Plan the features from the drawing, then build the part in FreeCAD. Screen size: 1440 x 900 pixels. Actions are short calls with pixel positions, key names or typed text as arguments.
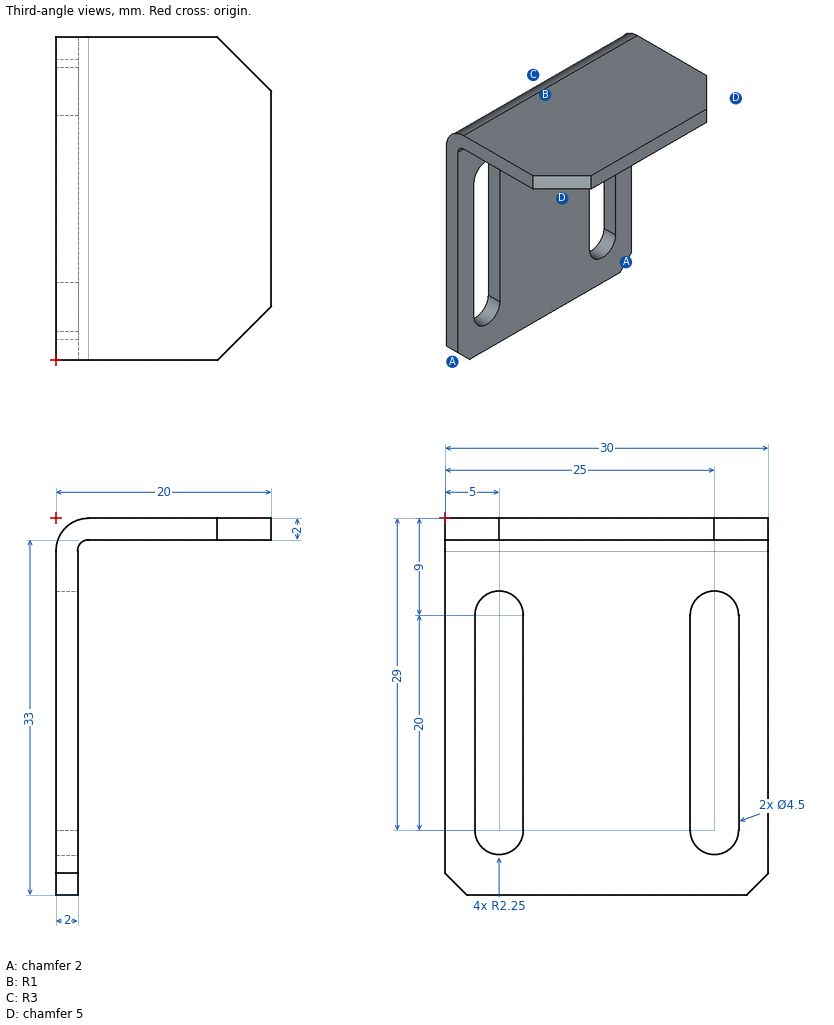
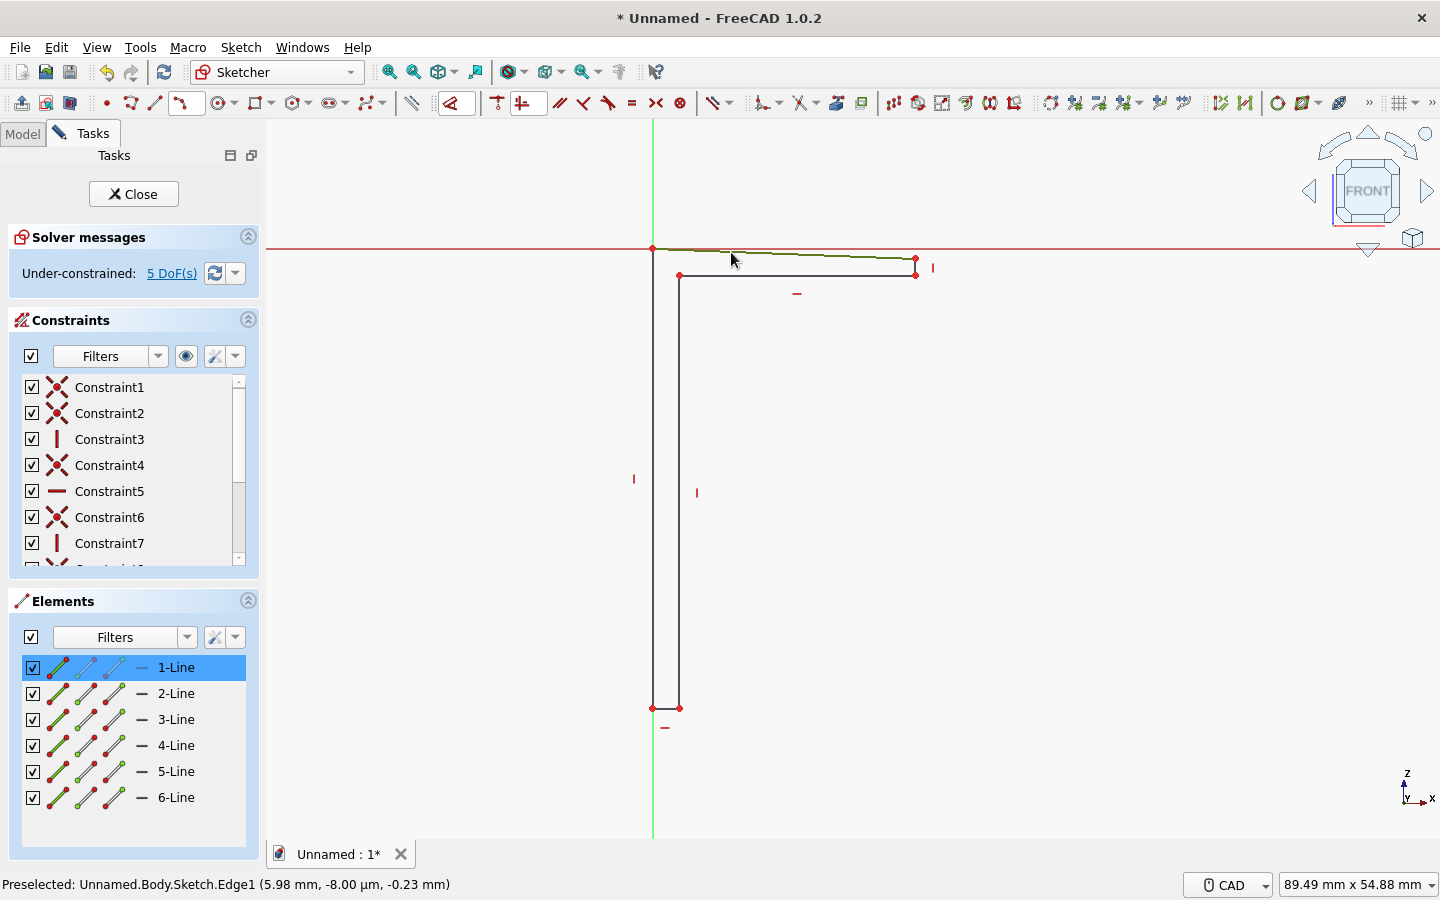
click(542, 104)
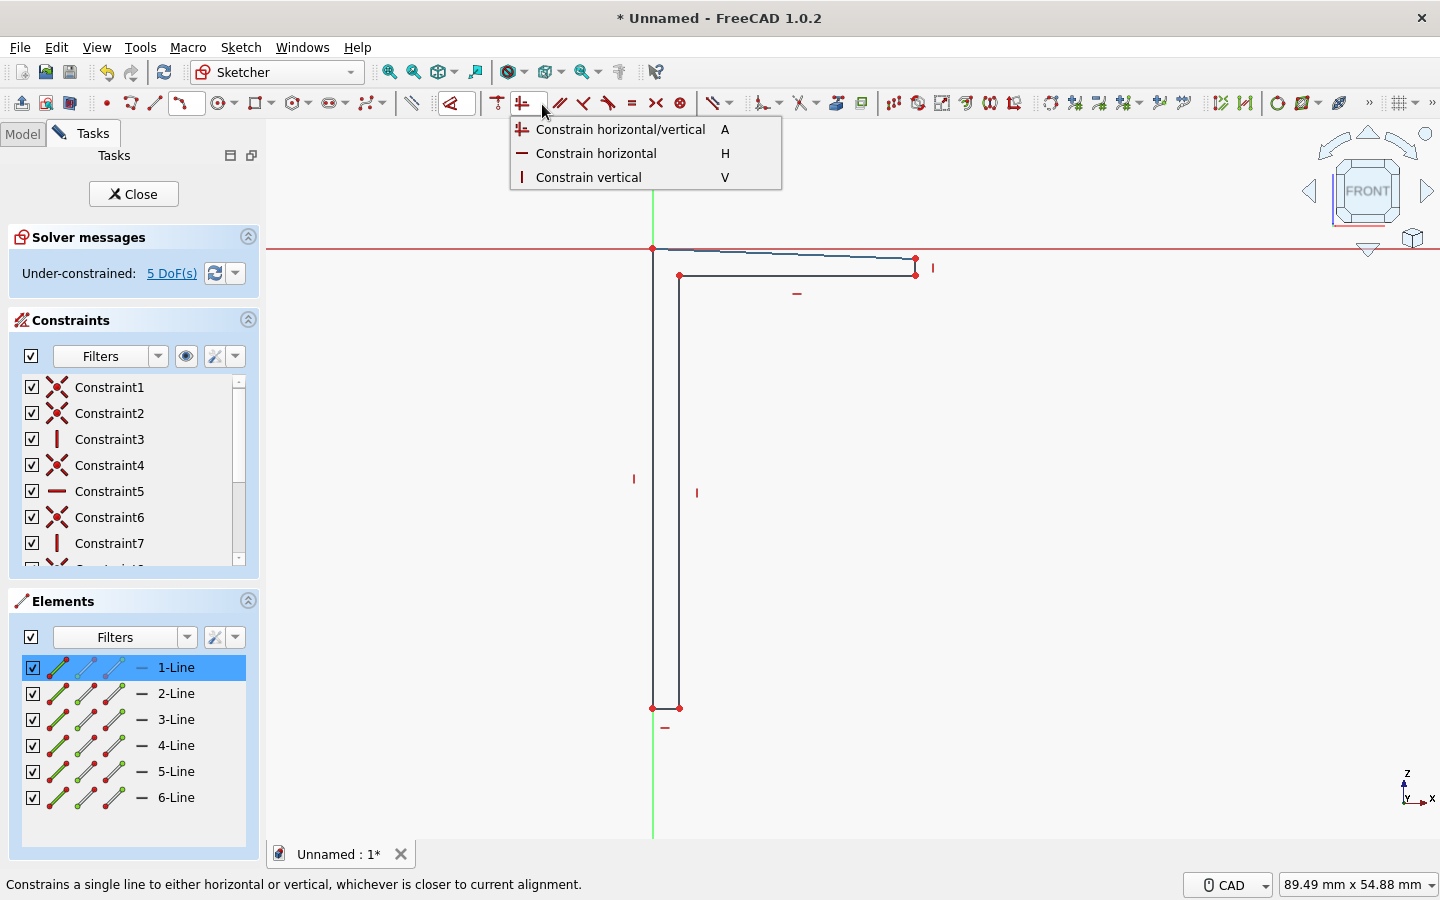
click(646, 153)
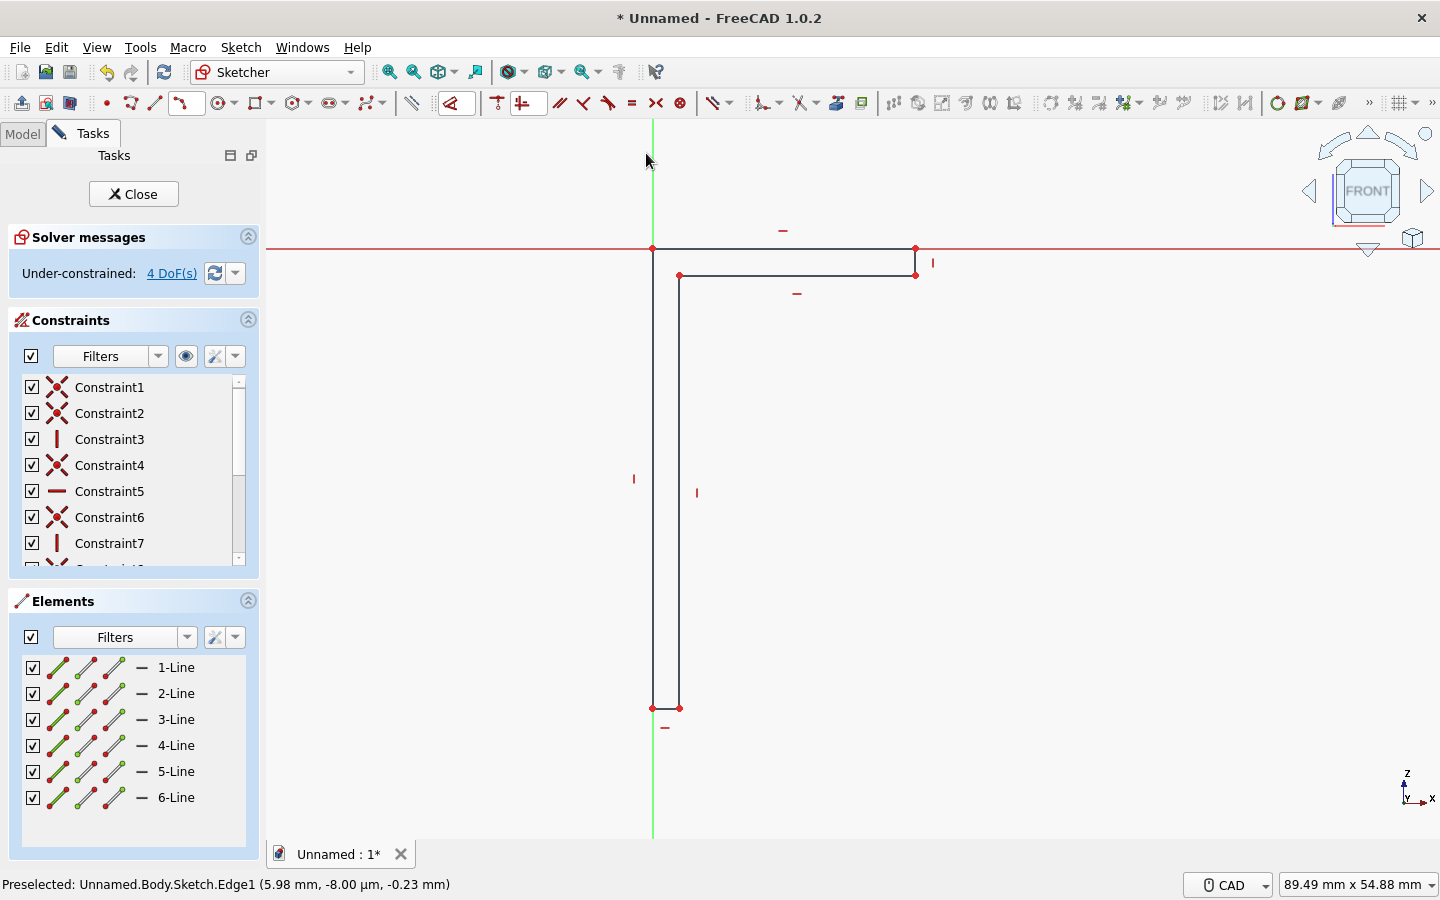
click(450, 104)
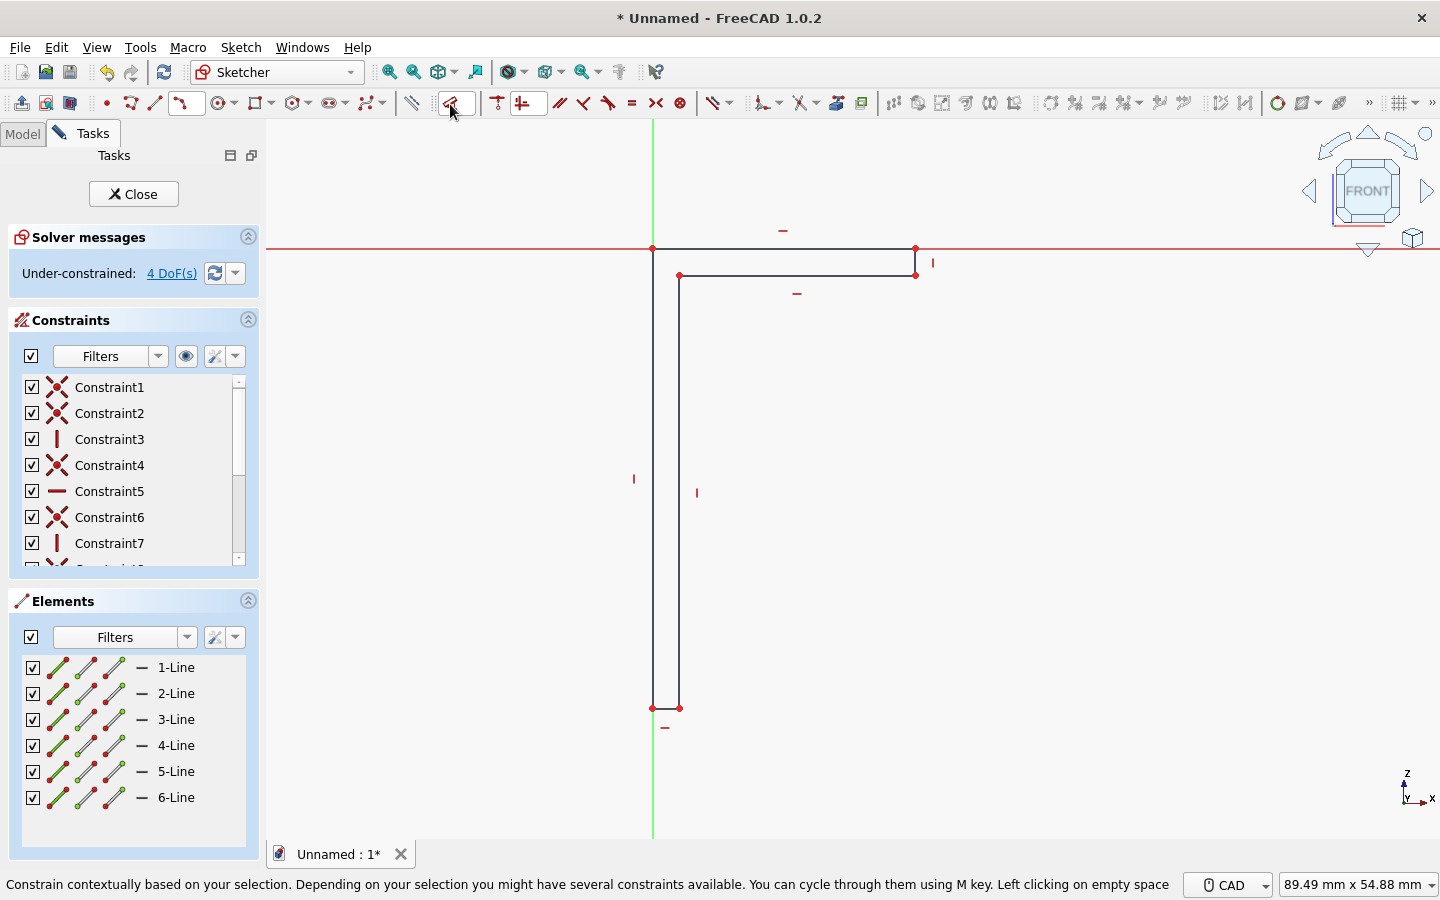
scroll(915, 260, up, 3)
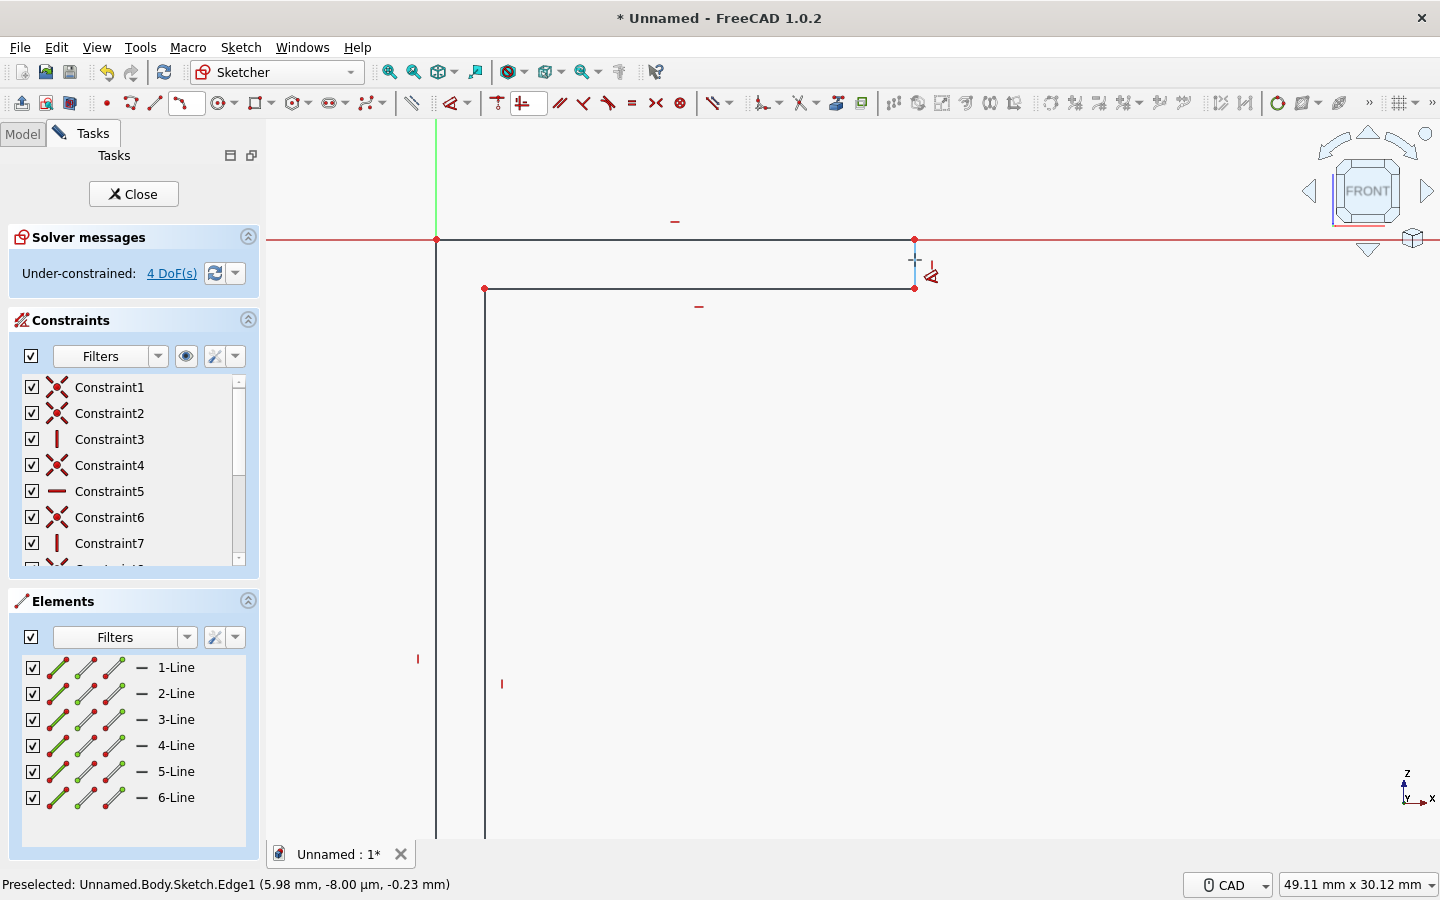
click(915, 259)
click(949, 264)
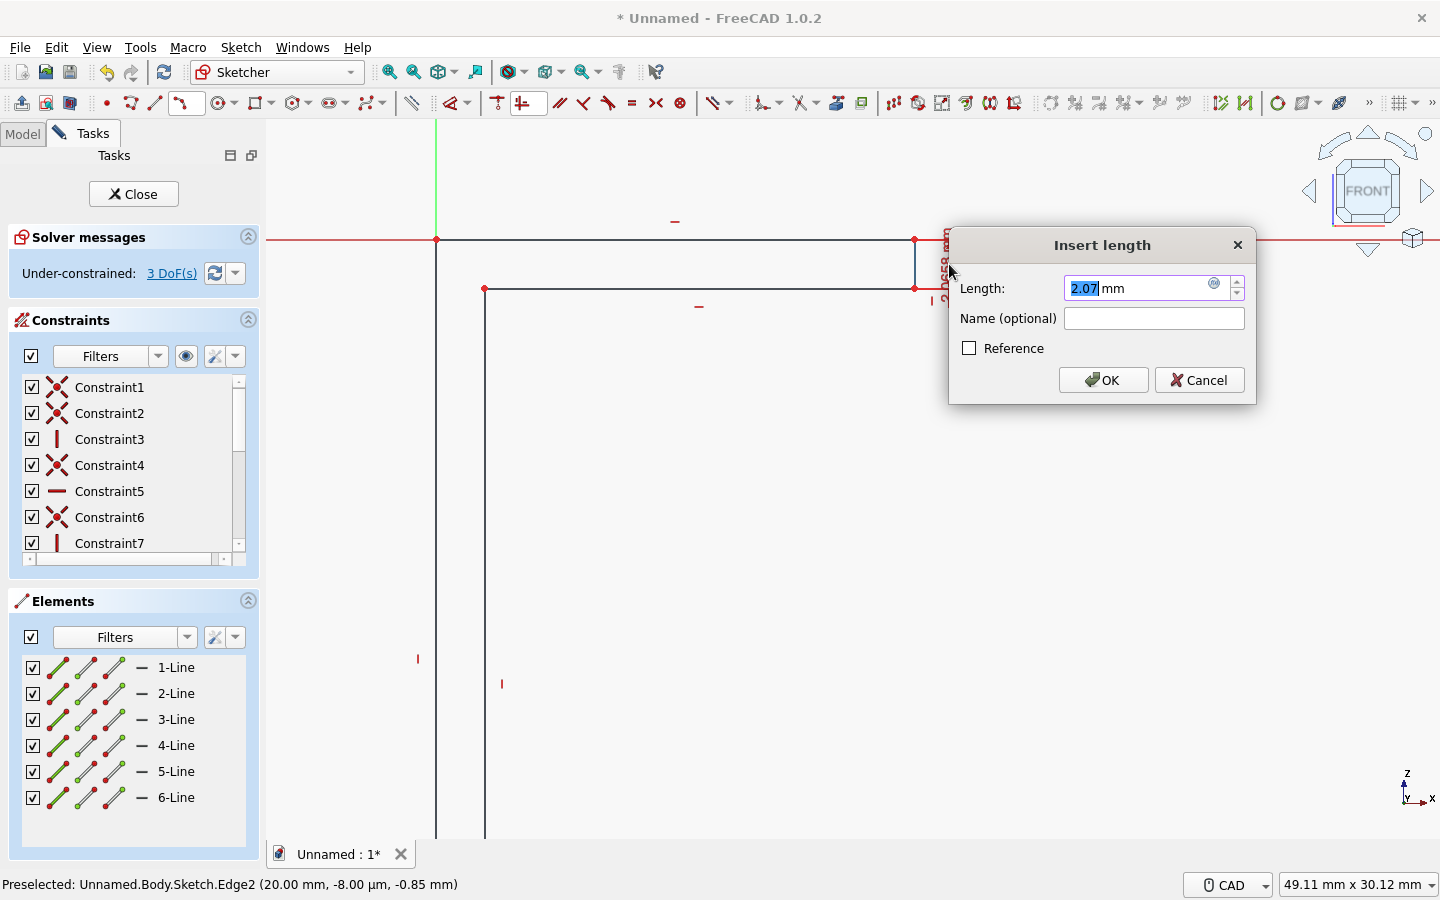
text(2)
key(Return)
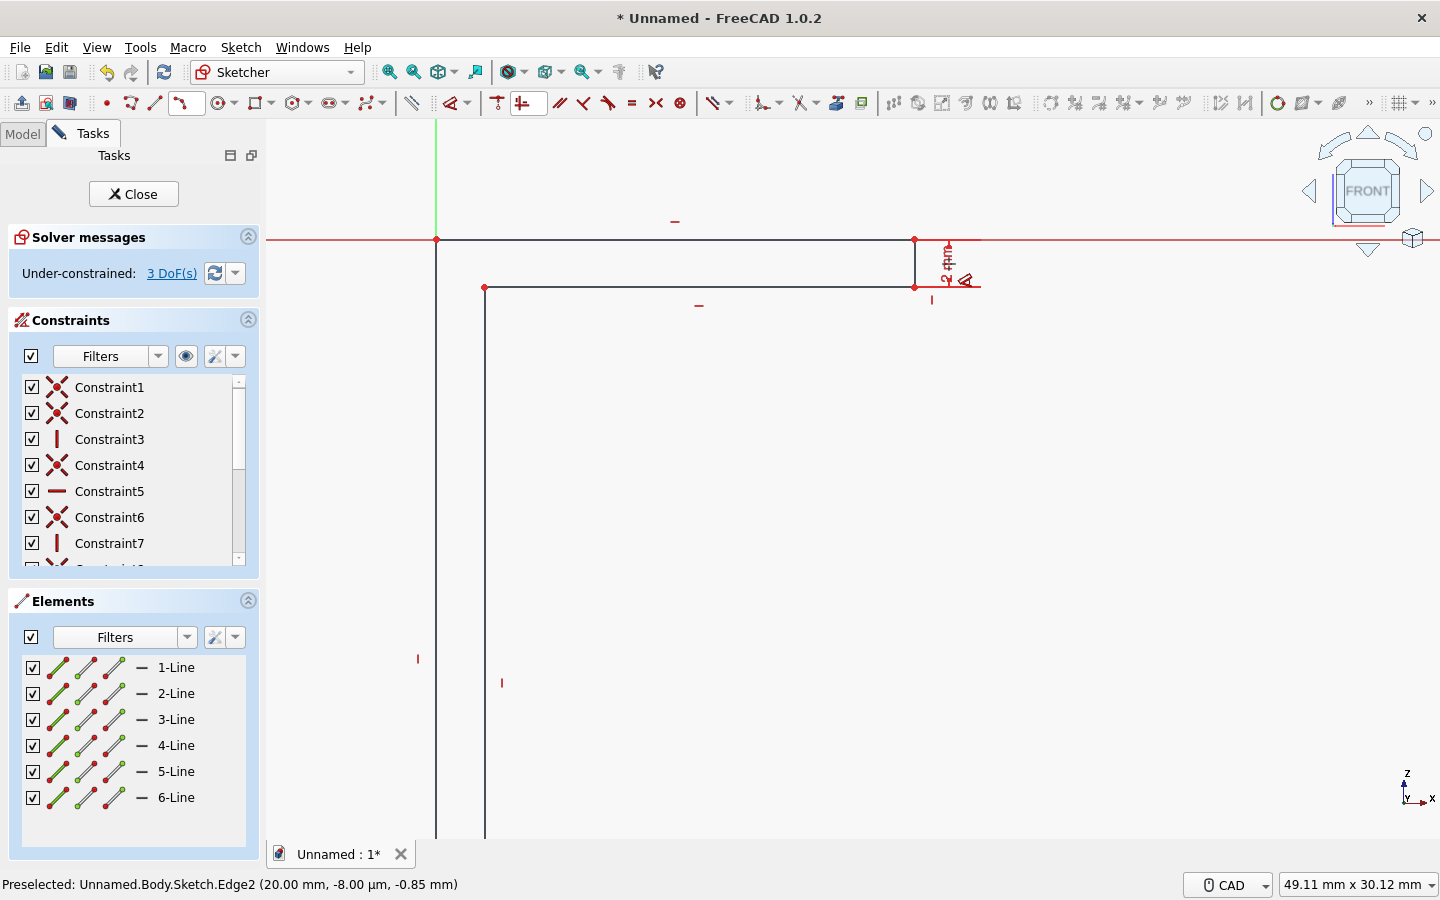
scroll(917, 261, down, 3)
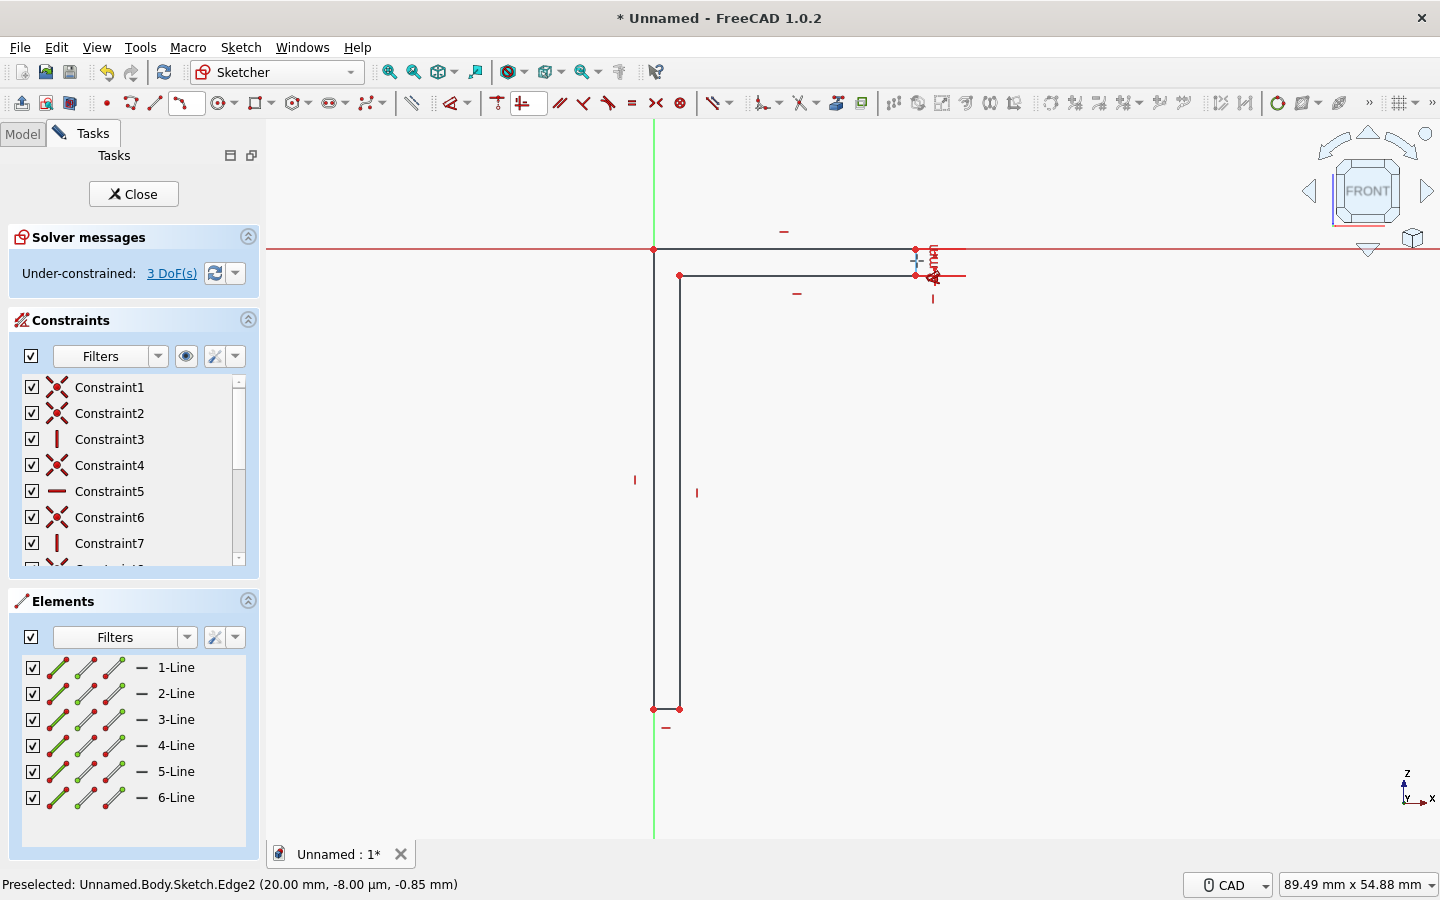
scroll(672, 709, up, 3)